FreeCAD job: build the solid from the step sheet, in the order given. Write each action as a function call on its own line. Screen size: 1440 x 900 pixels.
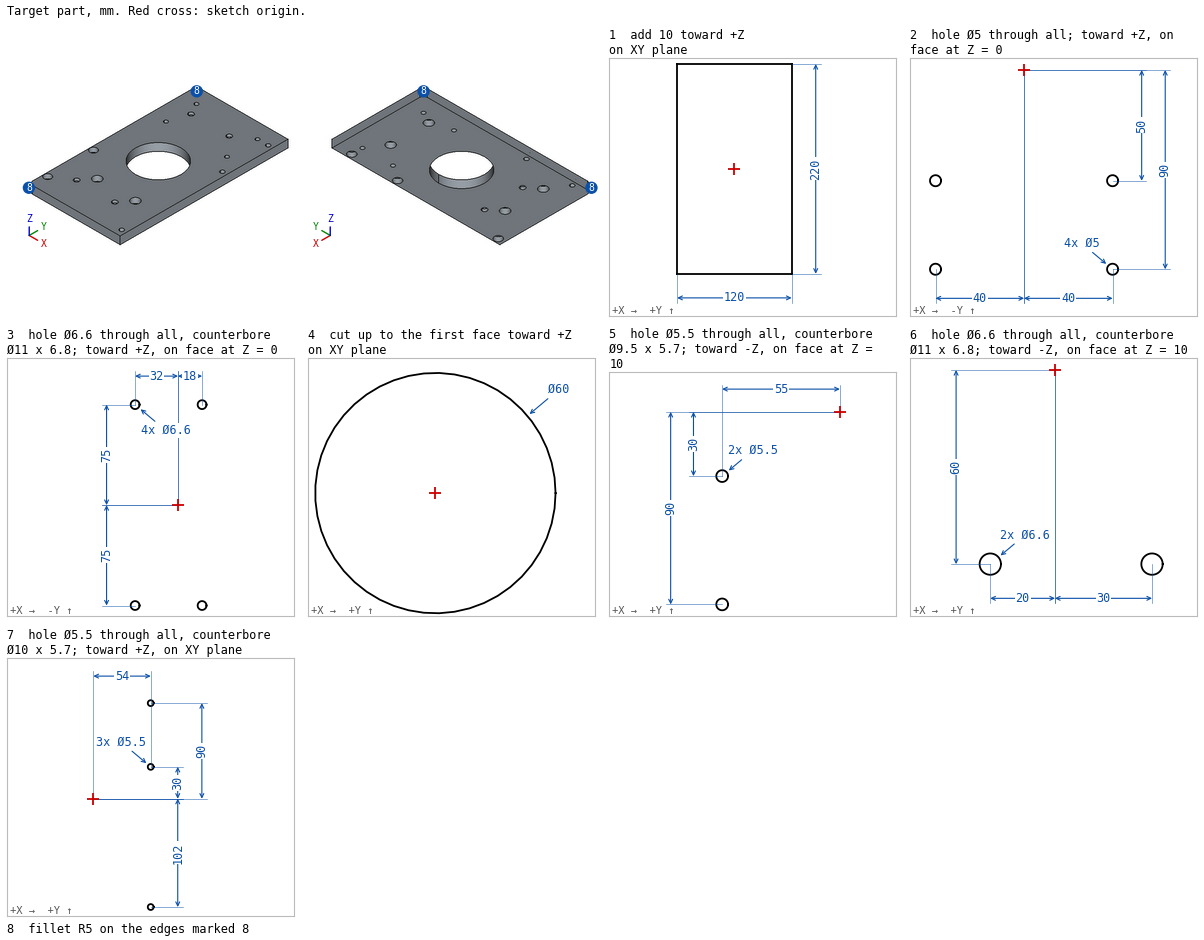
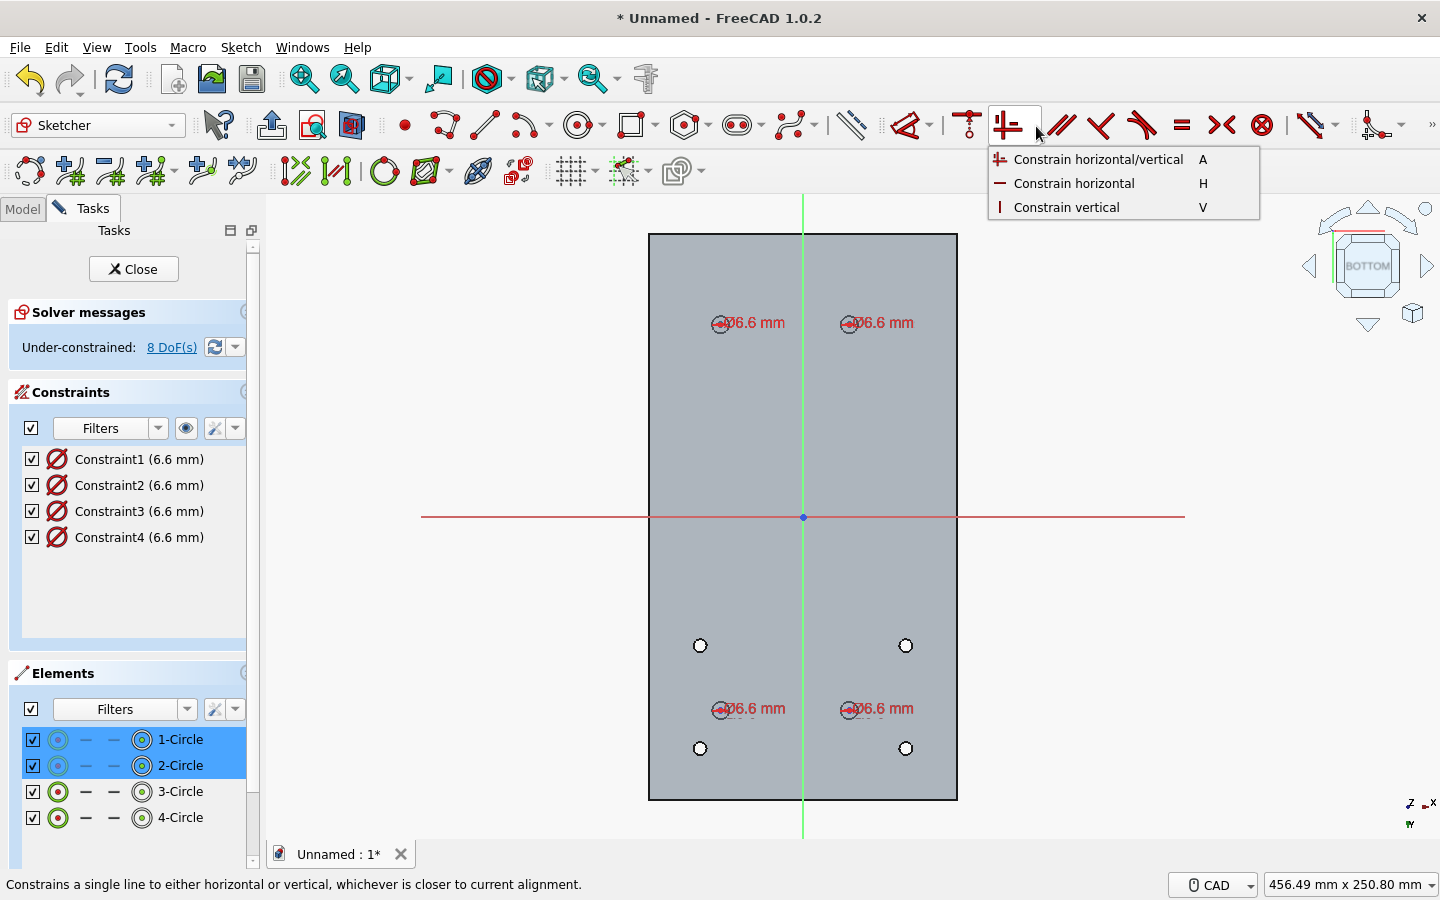
click(1124, 183)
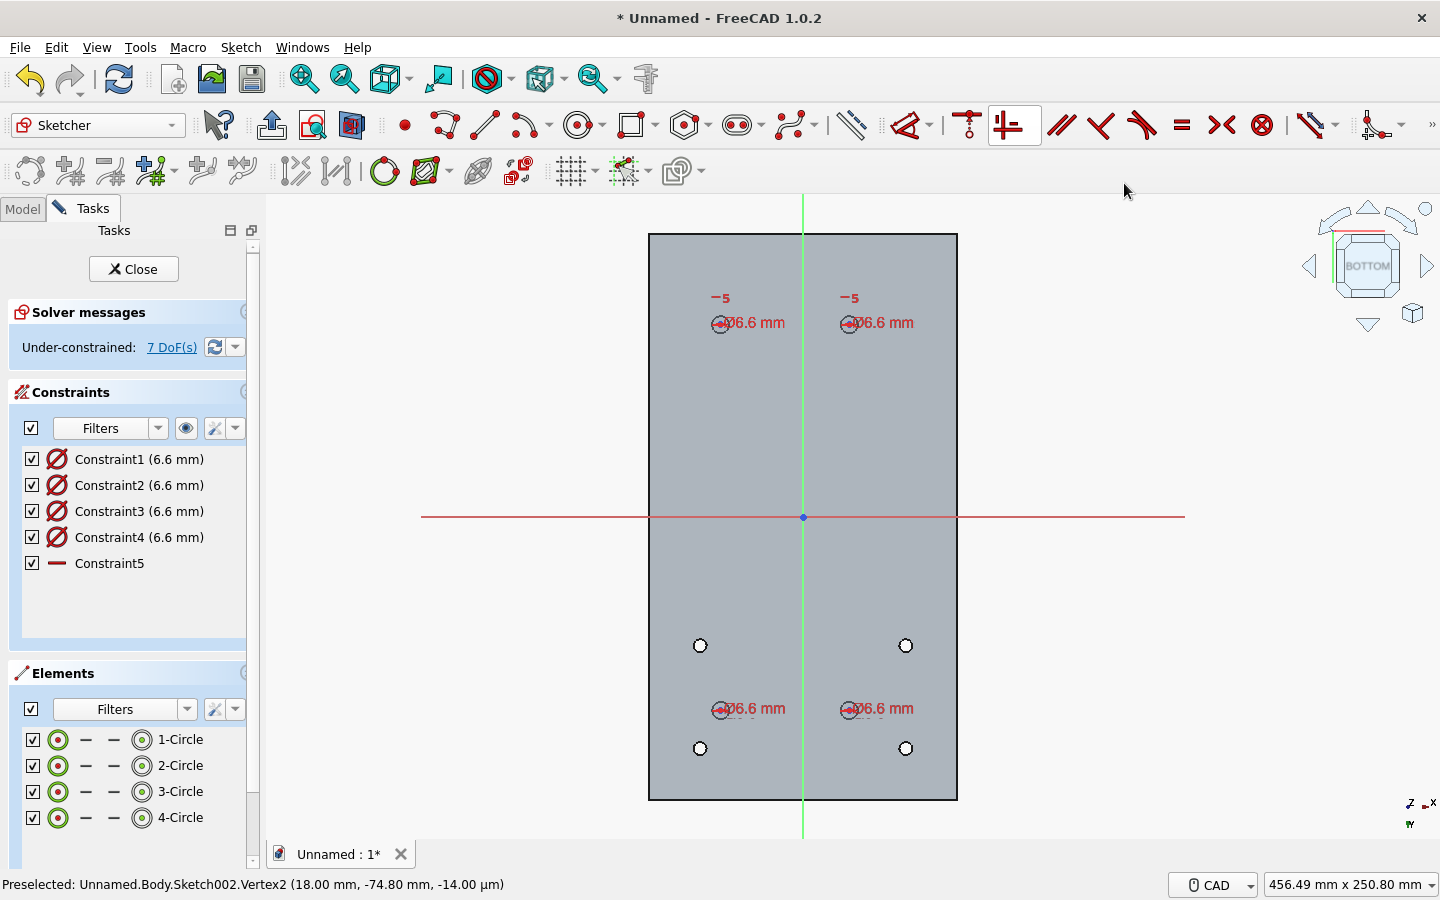
click(721, 325)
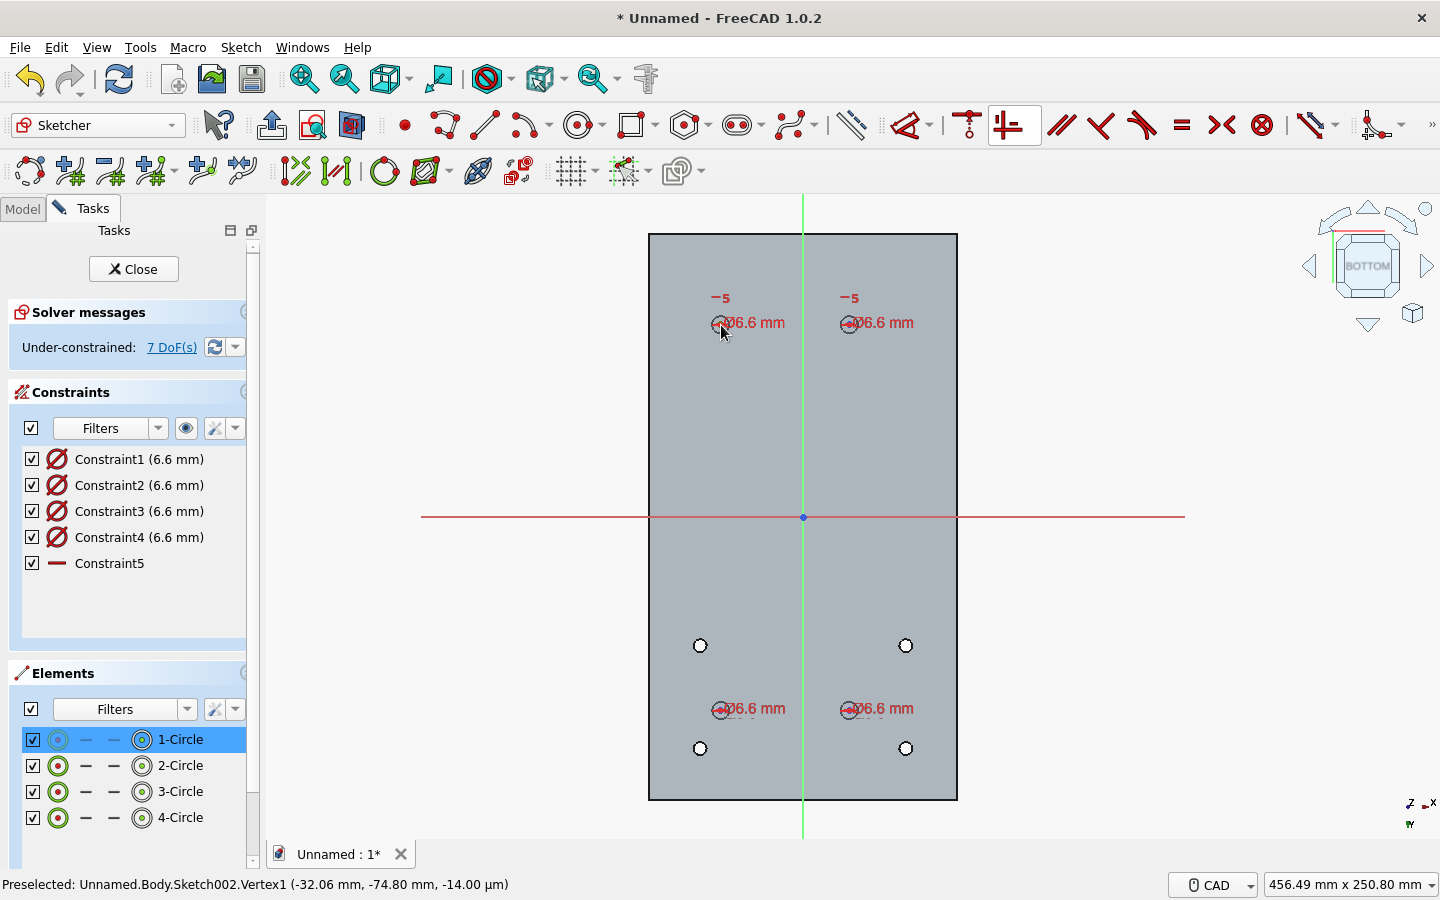
click(721, 711)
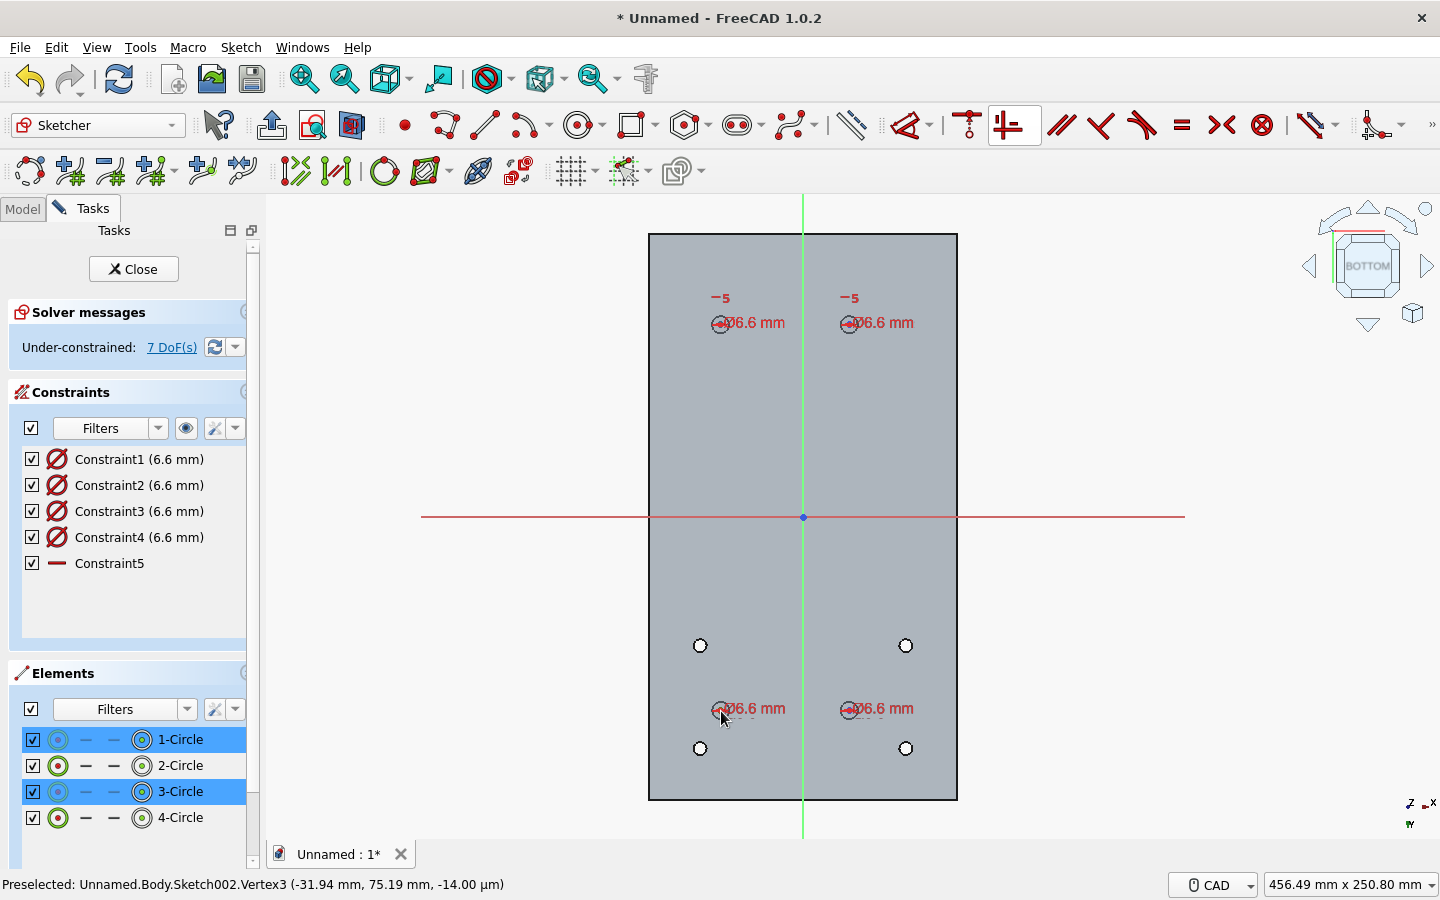
key(v)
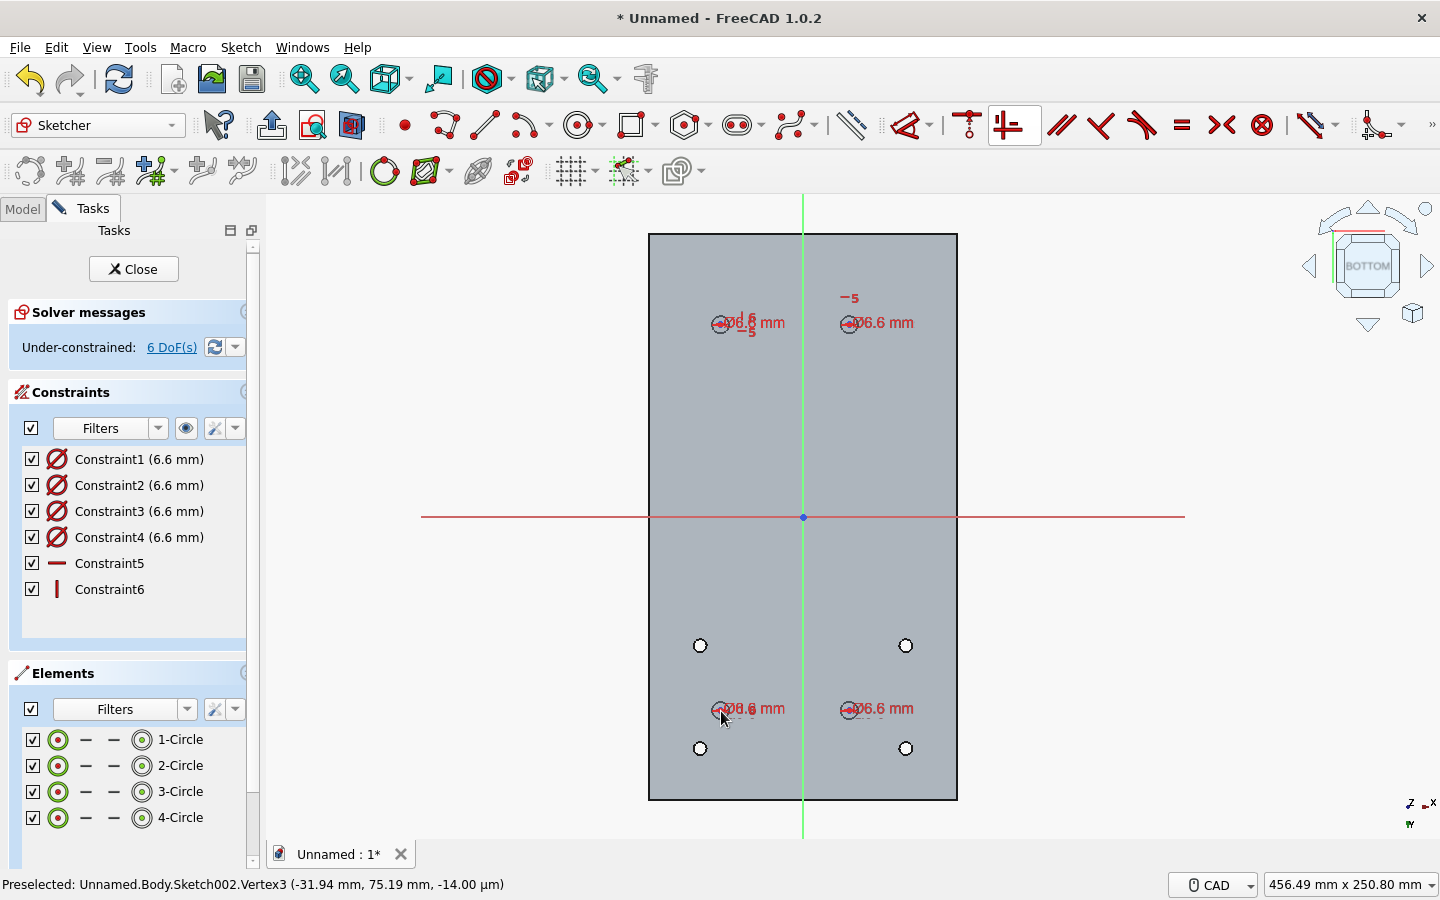
click(849, 325)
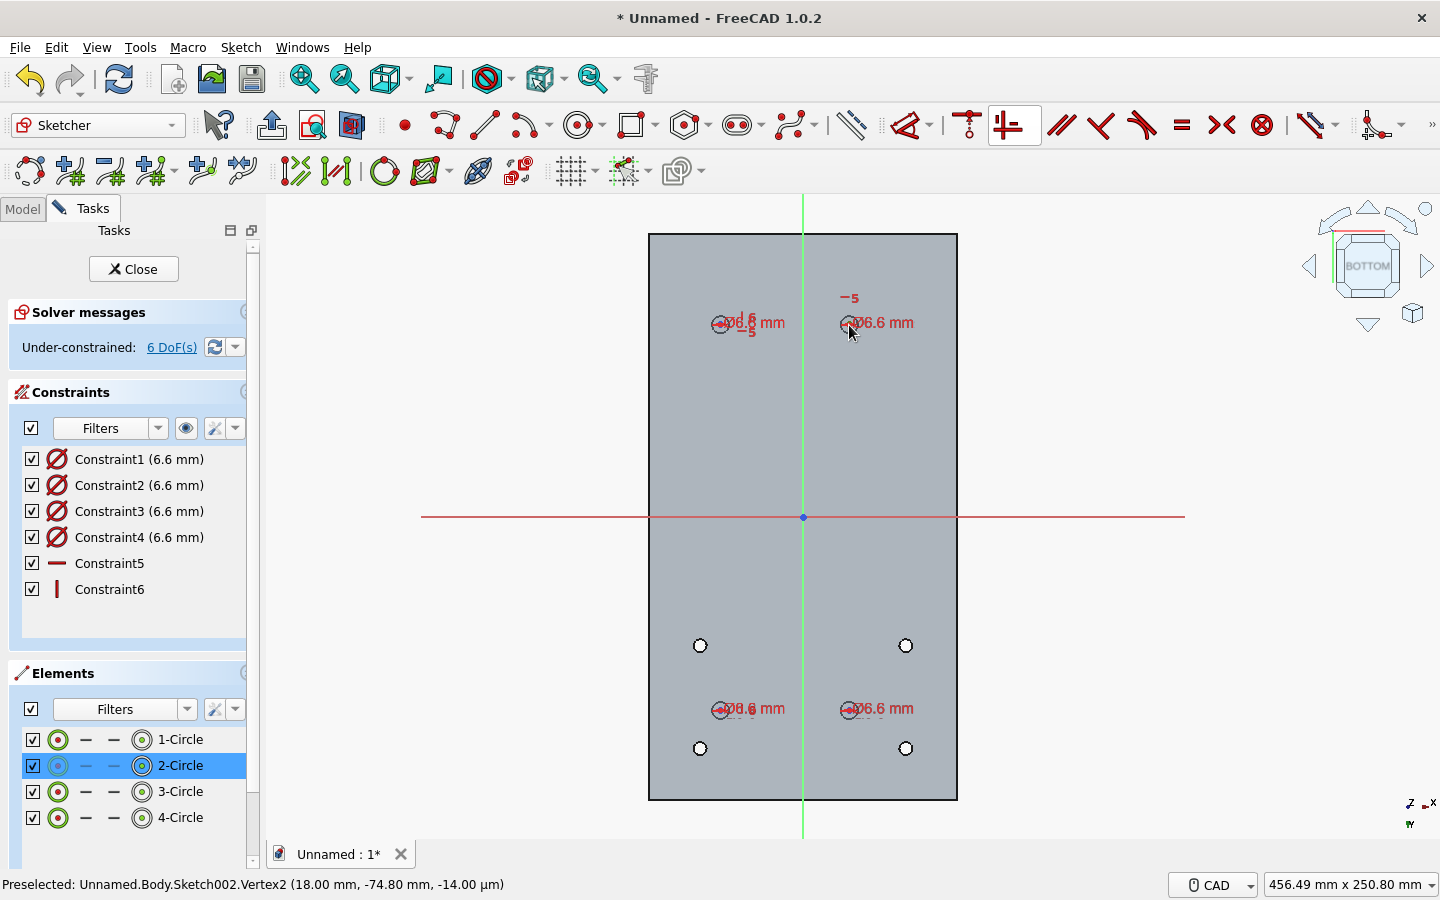
click(849, 711)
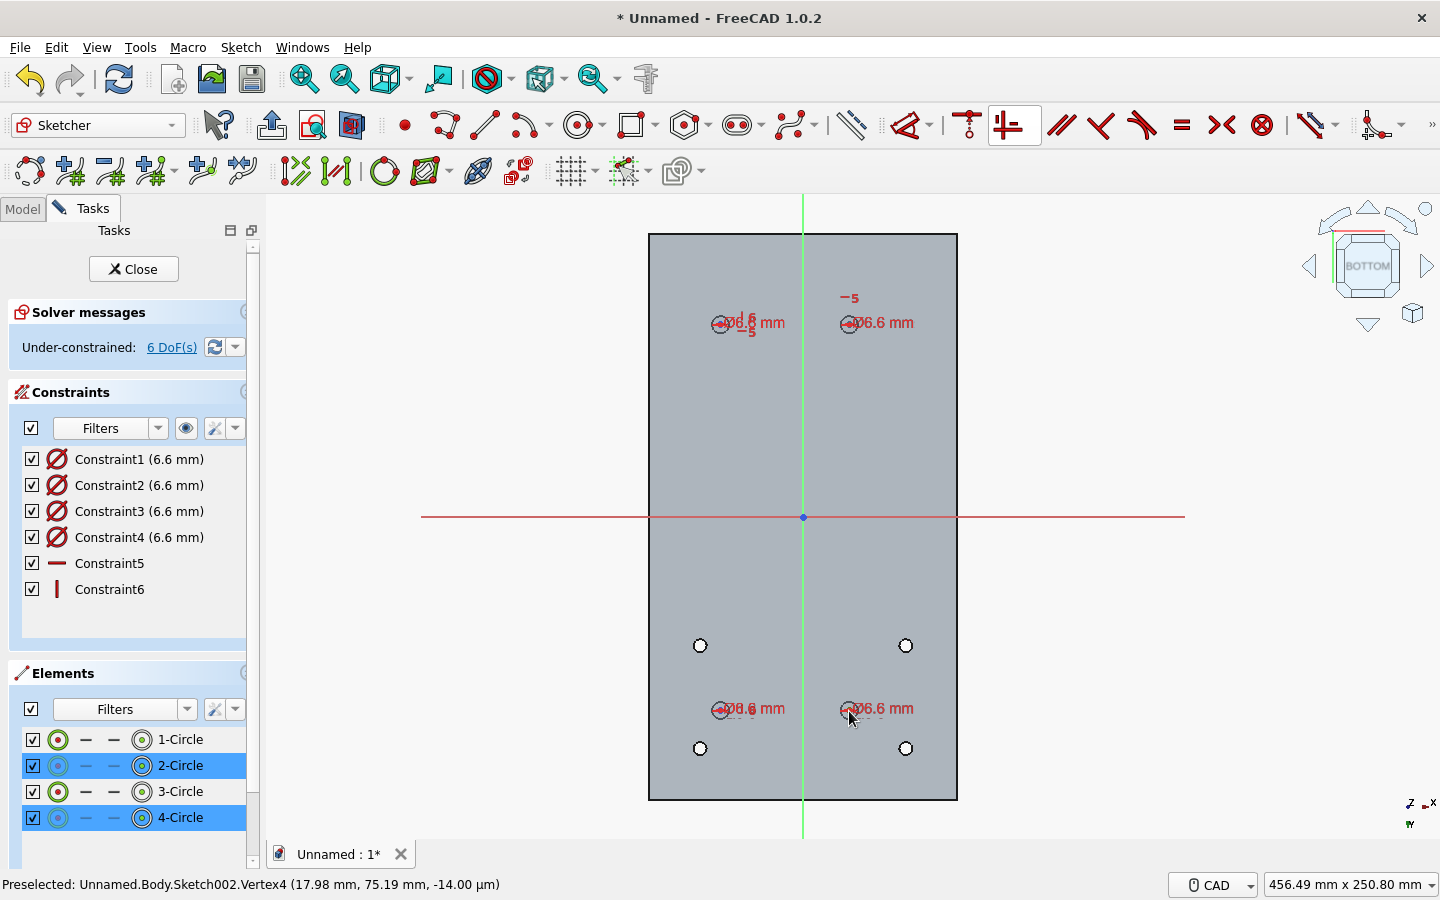
key(v)